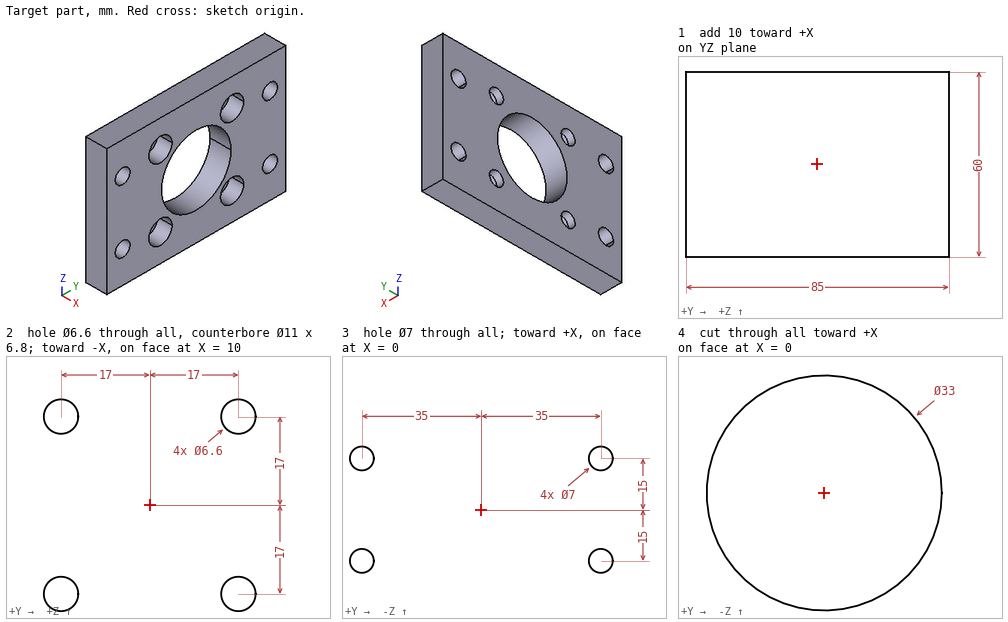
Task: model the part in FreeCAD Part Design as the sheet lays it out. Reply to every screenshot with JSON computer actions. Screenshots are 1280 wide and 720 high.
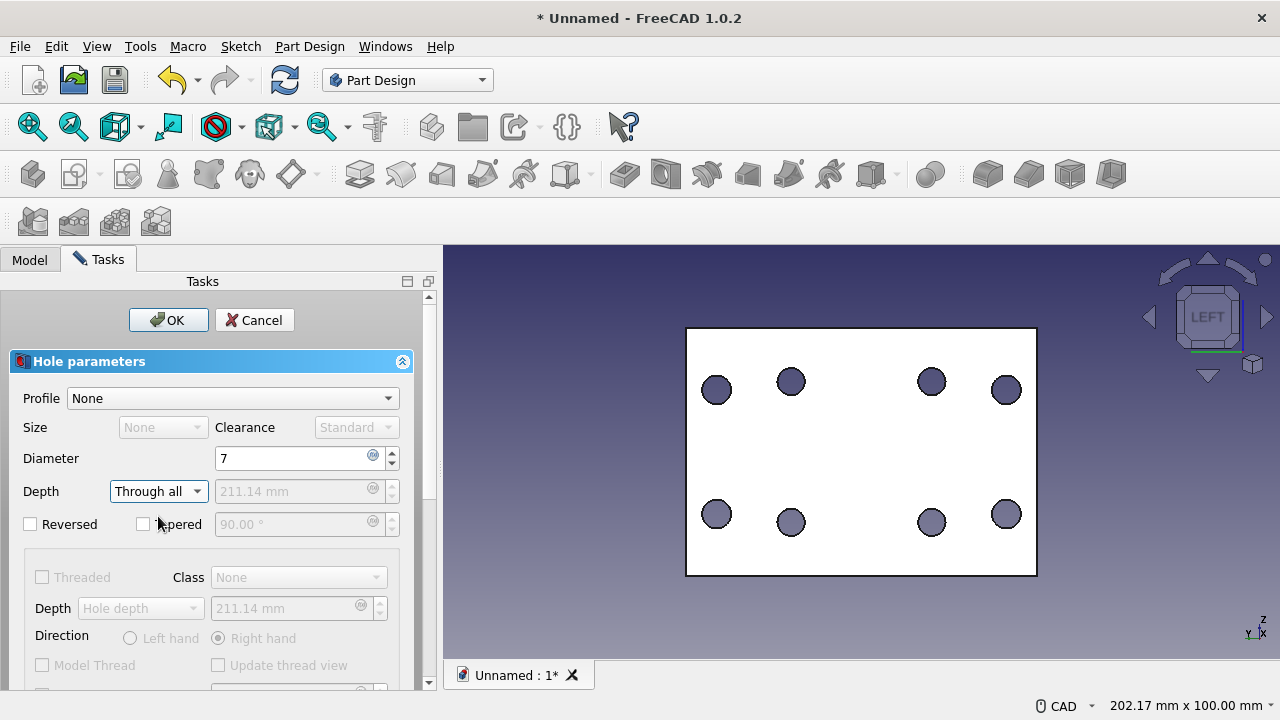
{"action": "left_click", "coordinate": [169, 320]}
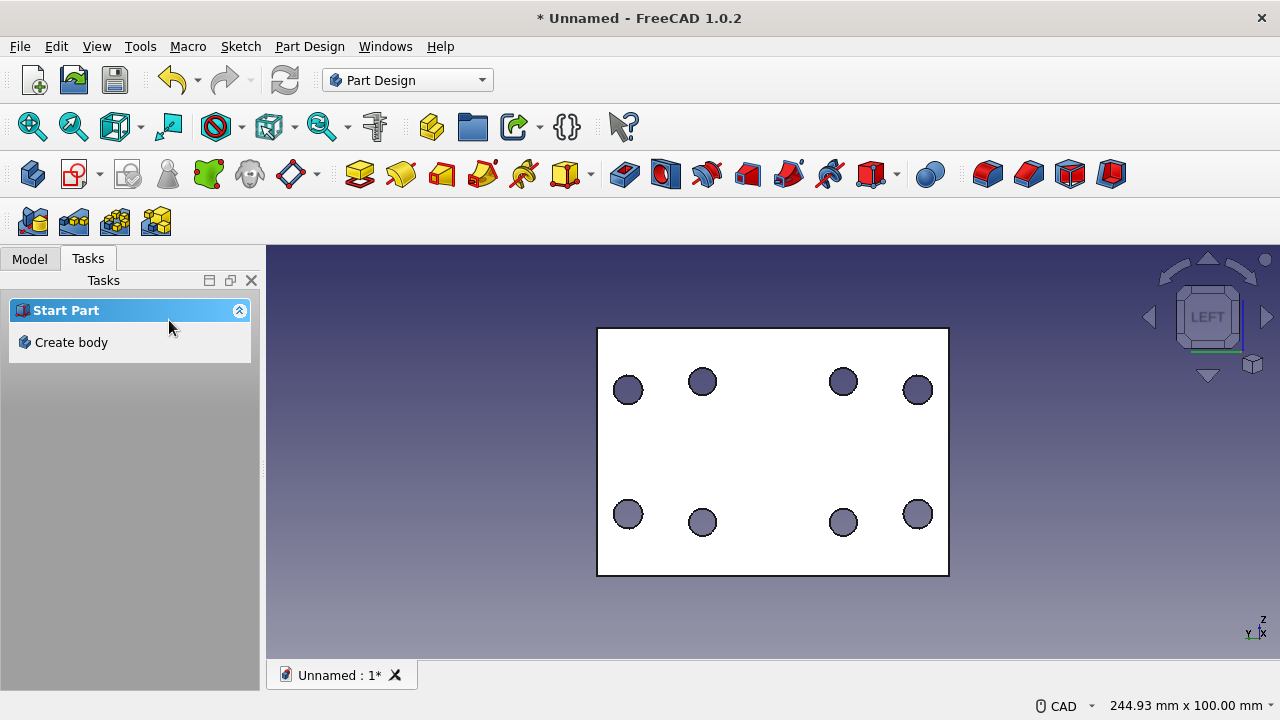
{"action": "left_click", "coordinate": [773, 451]}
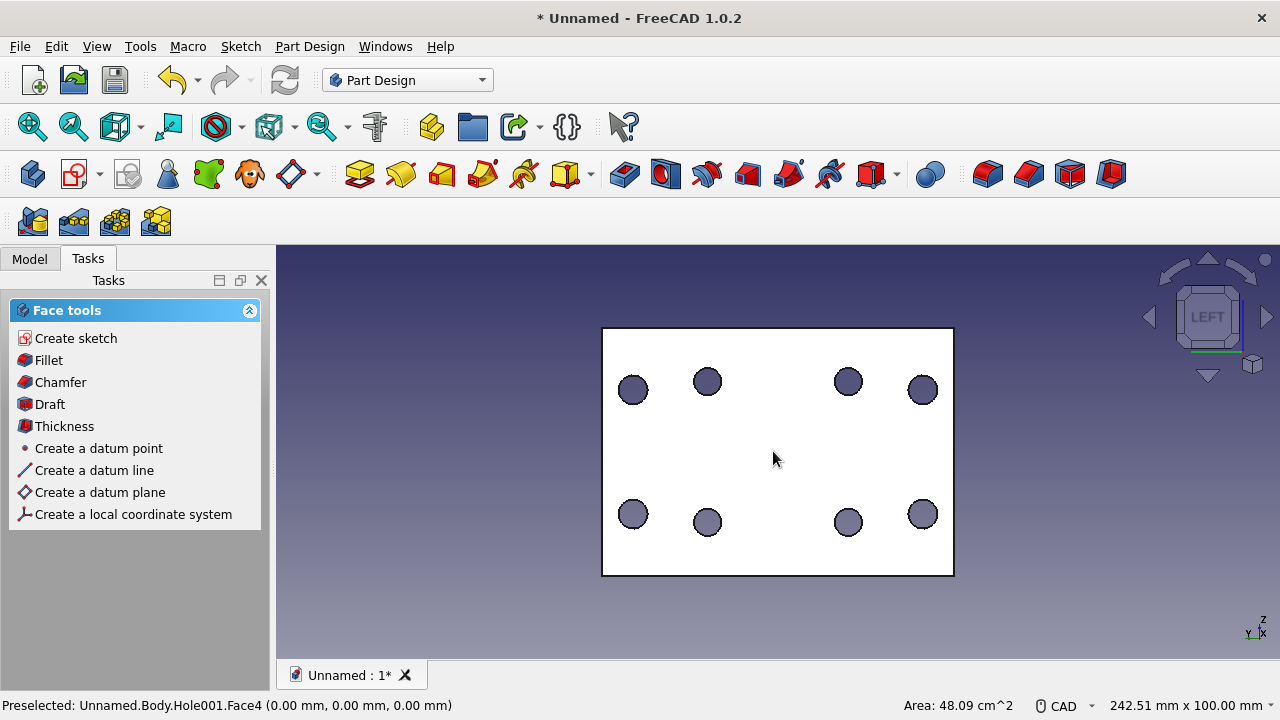
{"action": "left_click", "coordinate": [74, 174]}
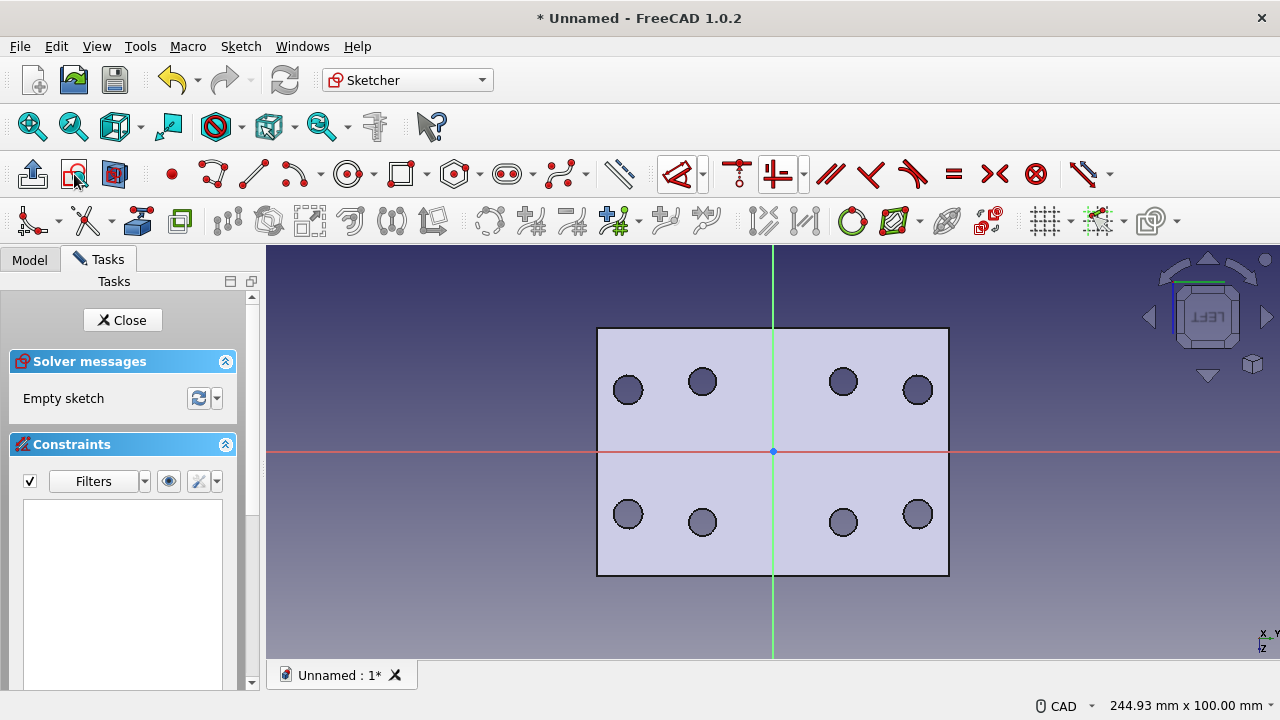
{"action": "scroll", "coordinate": [856, 452], "scroll_direction": "up", "scroll_amount": 3}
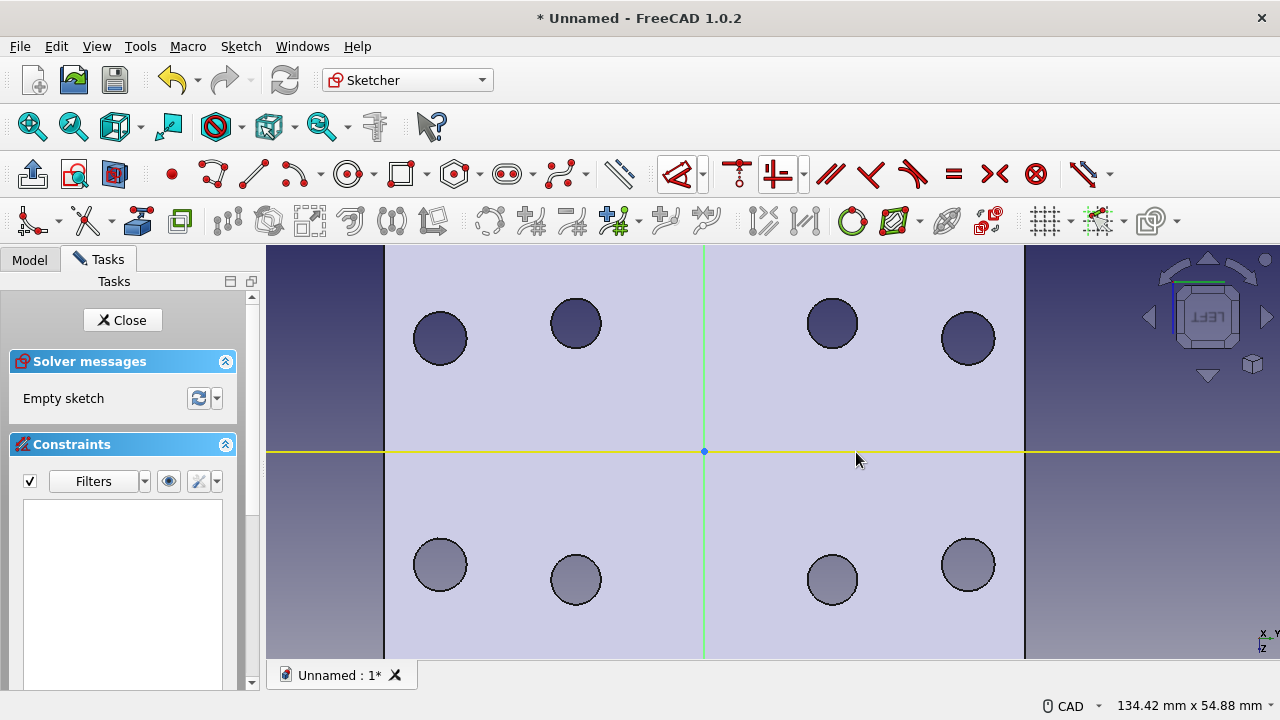
{"action": "key", "text": "g c"}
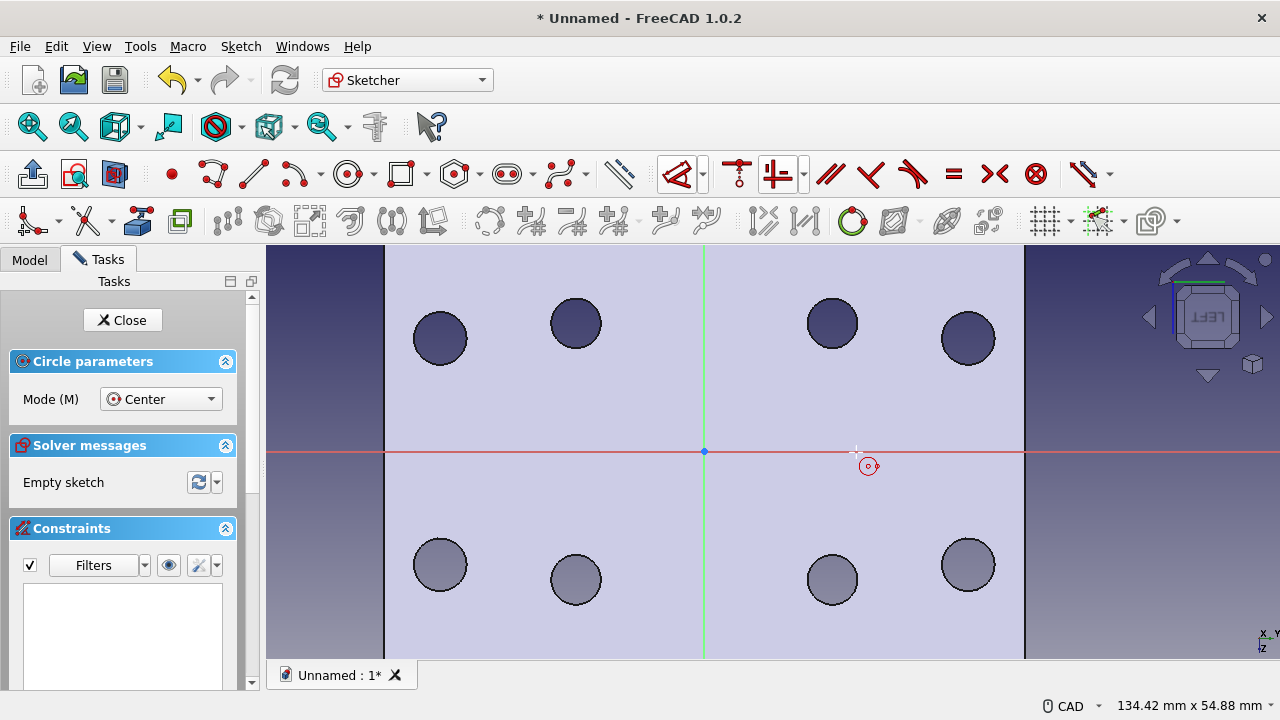
{"action": "left_click", "coordinate": [704, 452]}
{"action": "left_click", "coordinate": [792, 364]}
{"action": "key", "text": "Escape"}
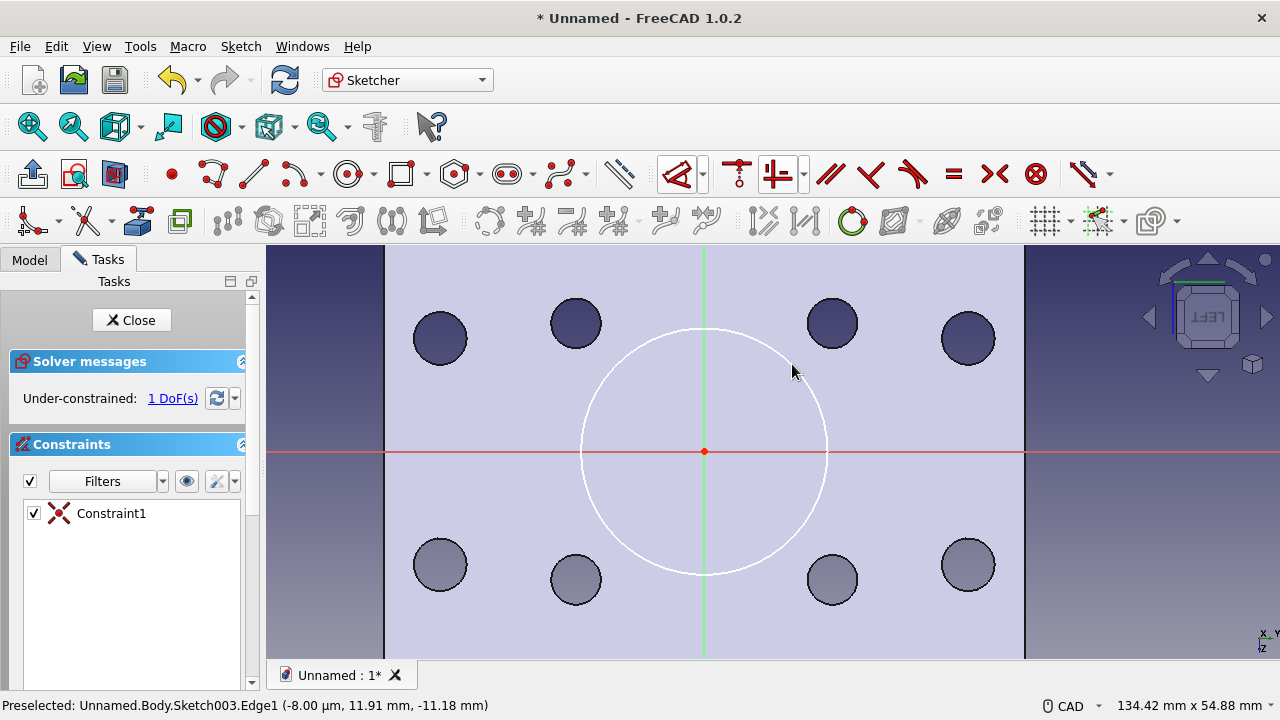
{"action": "left_click", "coordinate": [791, 364]}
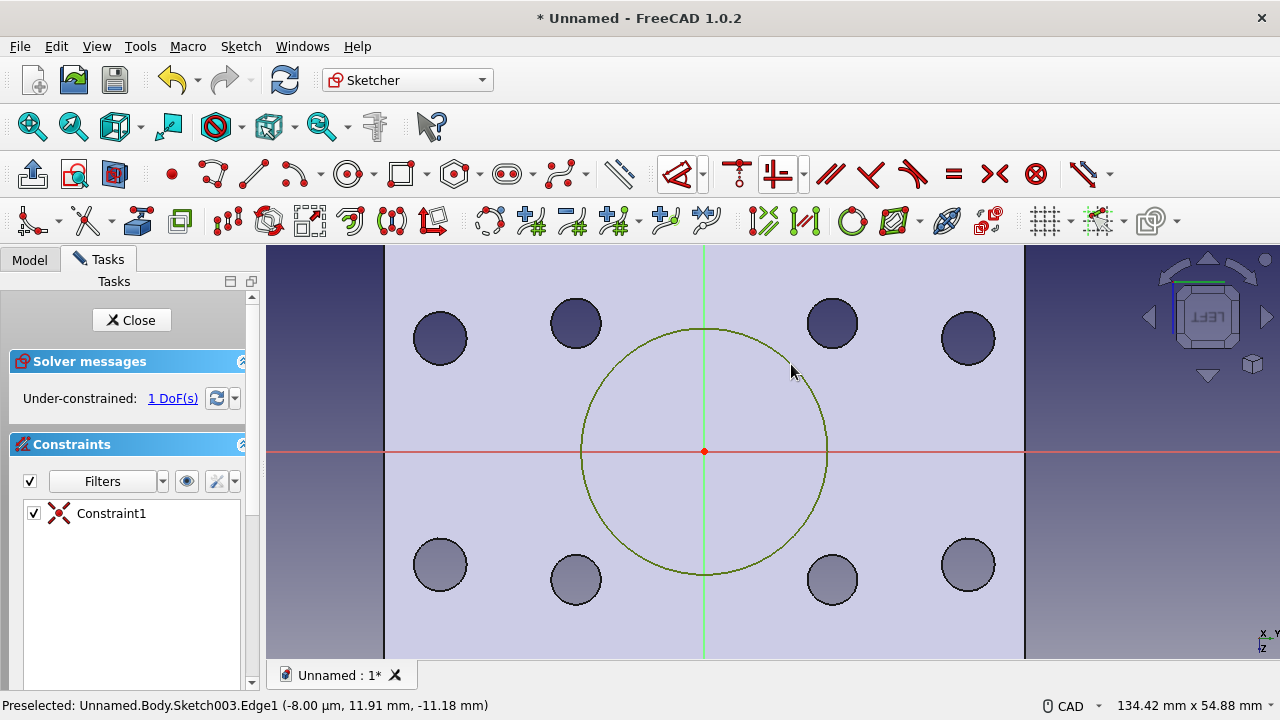
{"action": "key", "text": "k o"}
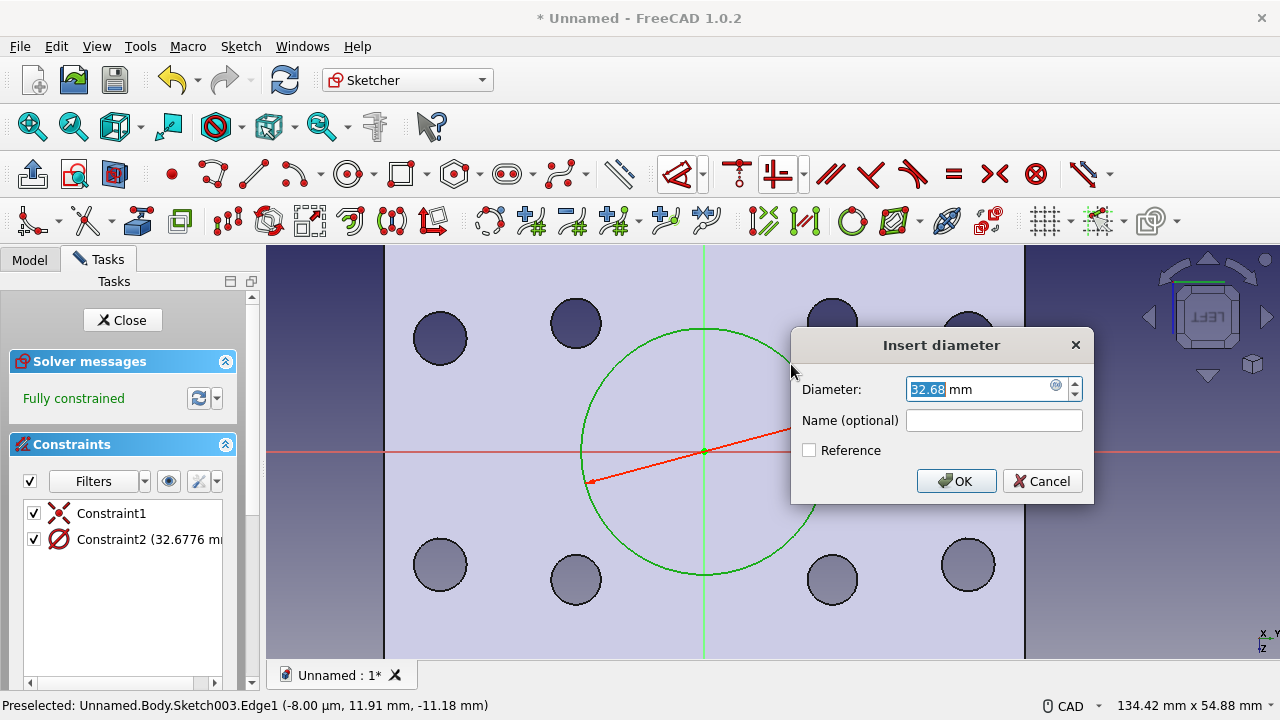
{"action": "type", "text": "33"}
{"action": "key", "text": "Return"}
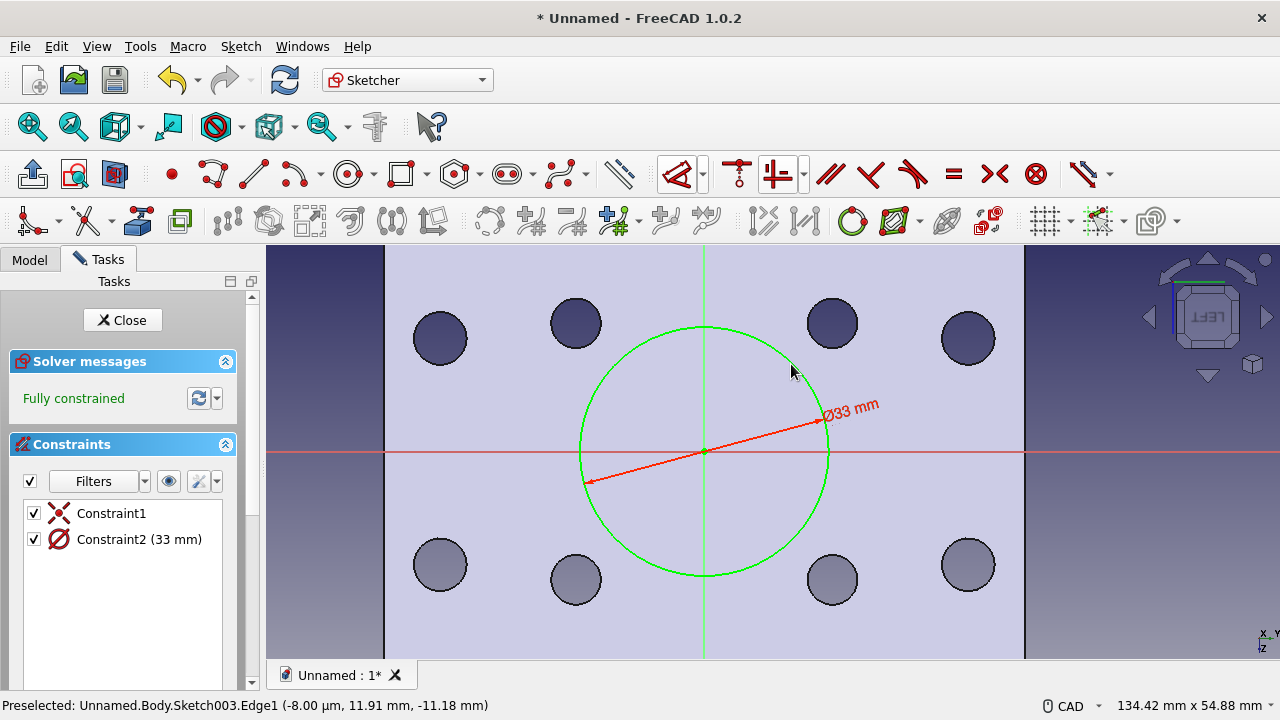
{"action": "left_click", "coordinate": [123, 320]}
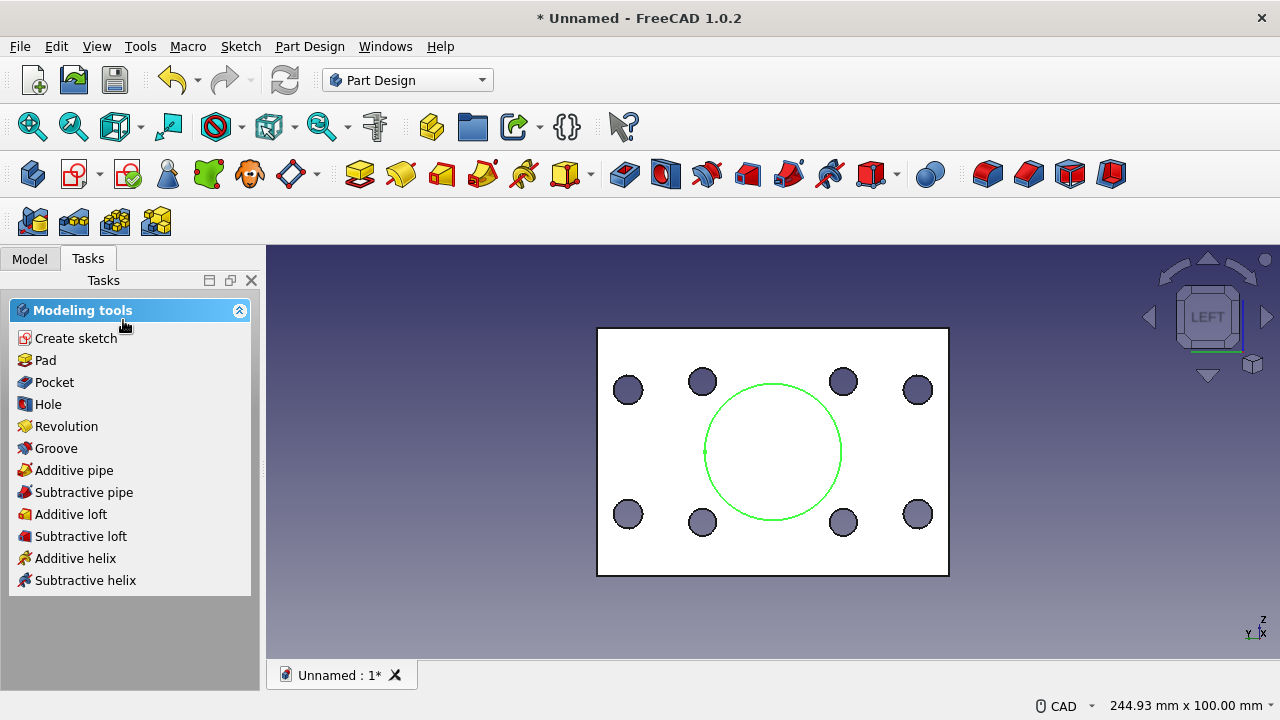
{"action": "left_click", "coordinate": [625, 174]}